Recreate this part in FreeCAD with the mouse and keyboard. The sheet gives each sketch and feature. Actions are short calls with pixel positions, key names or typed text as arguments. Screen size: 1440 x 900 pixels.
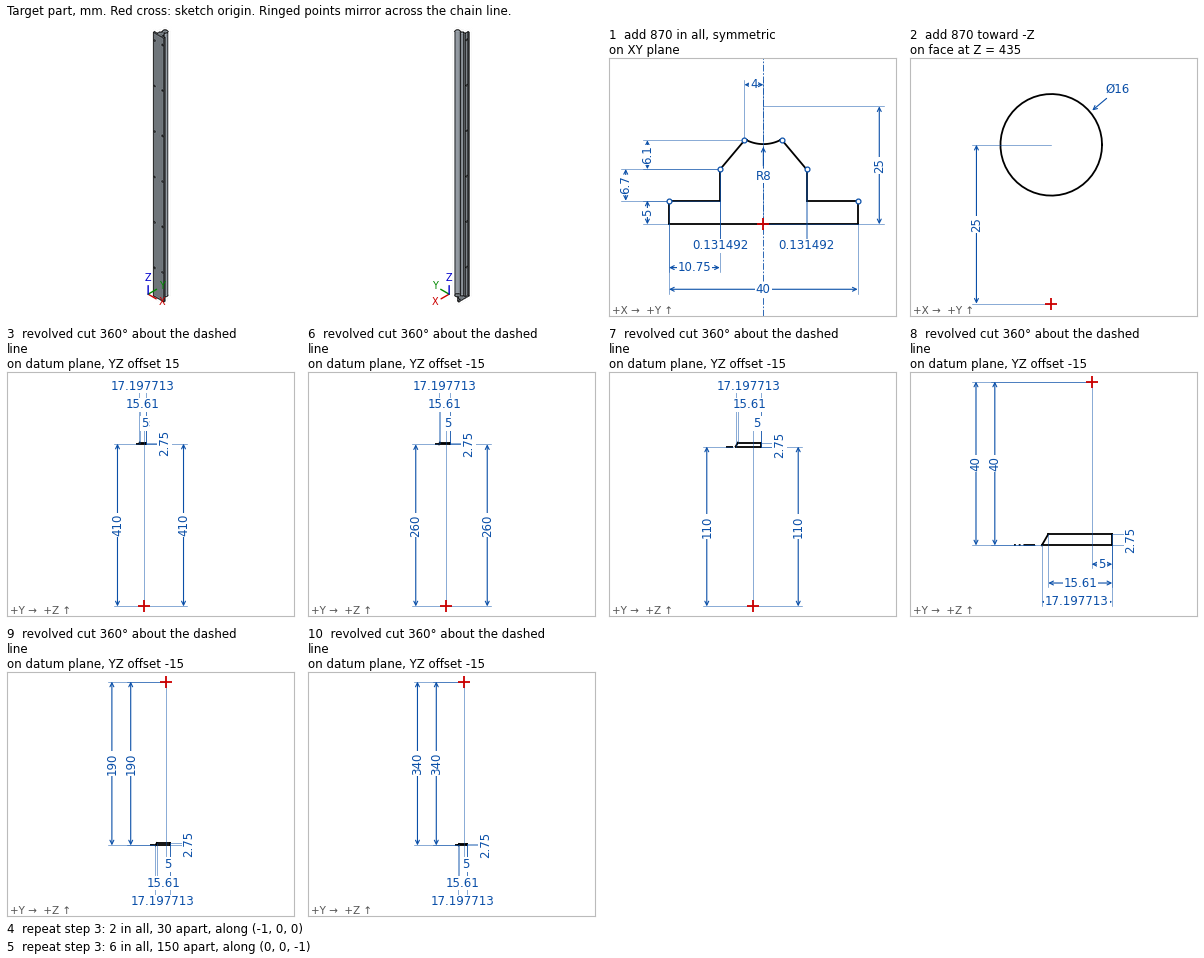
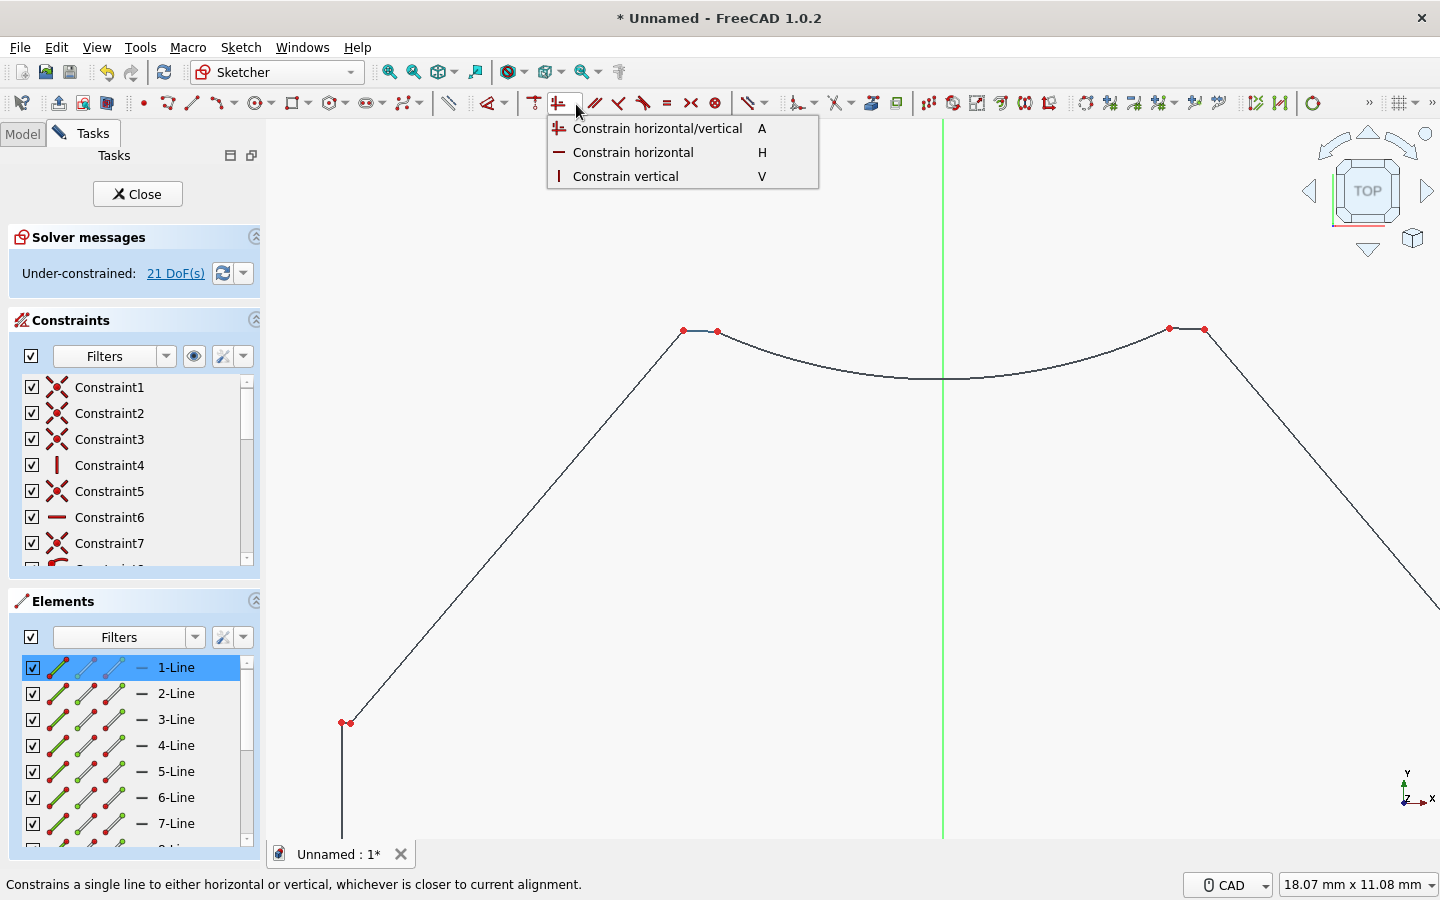
click(683, 152)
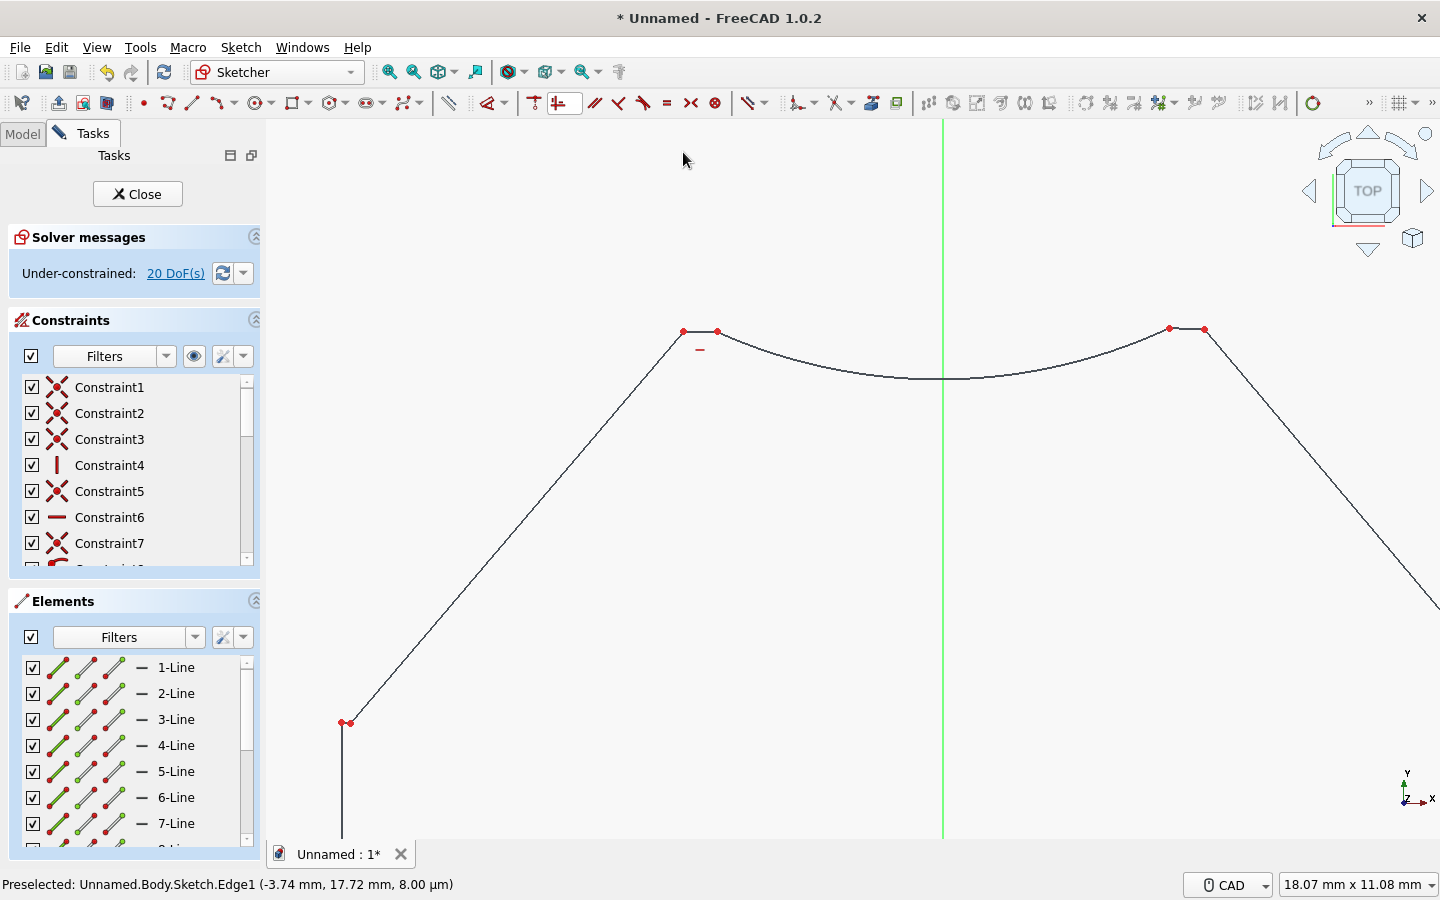
scroll(346, 723, up, 6)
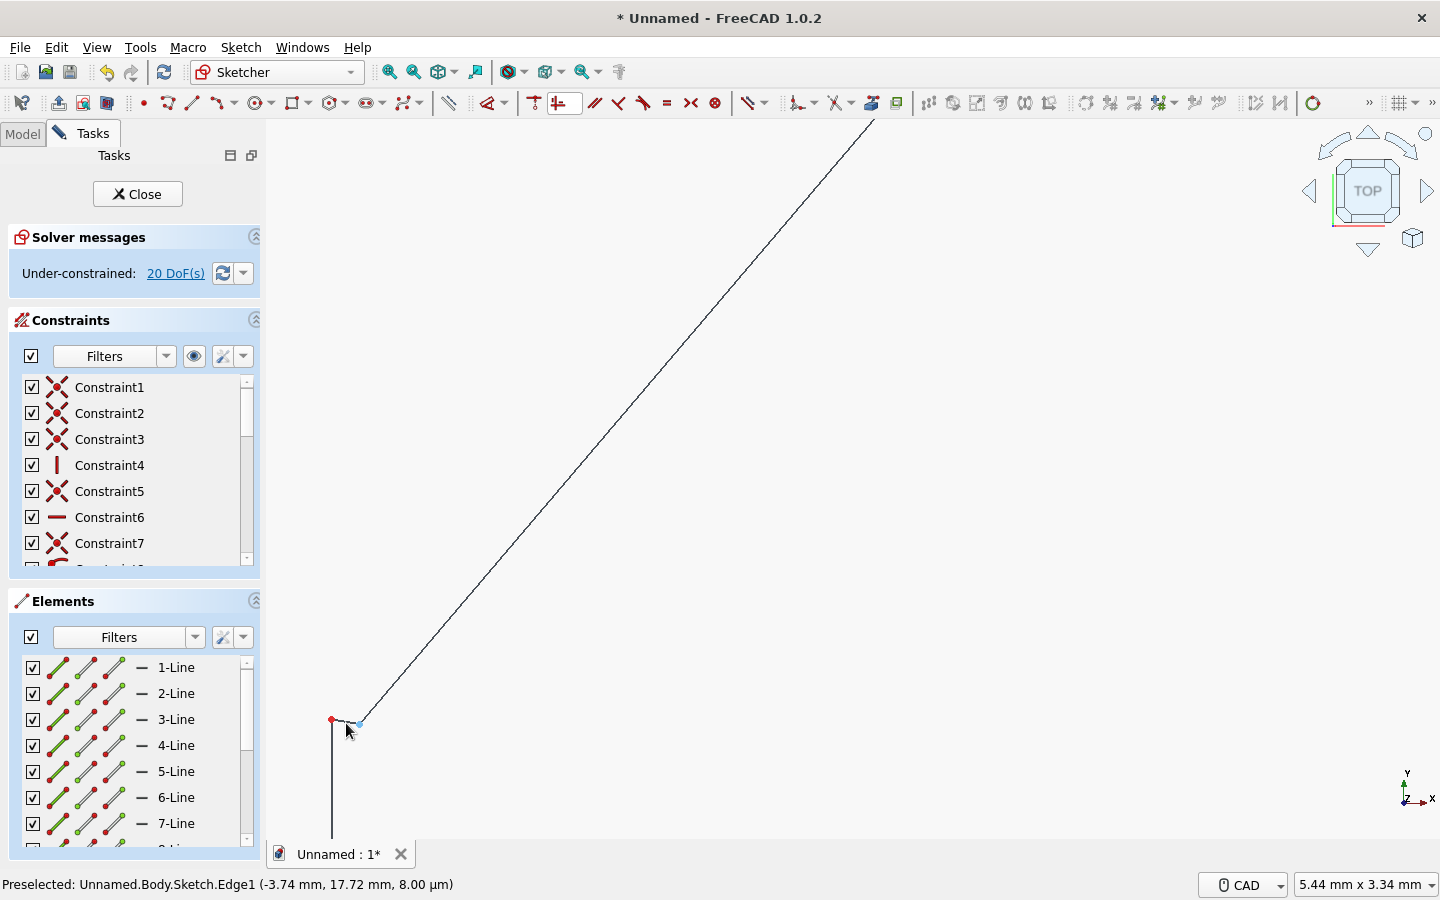
click(346, 722)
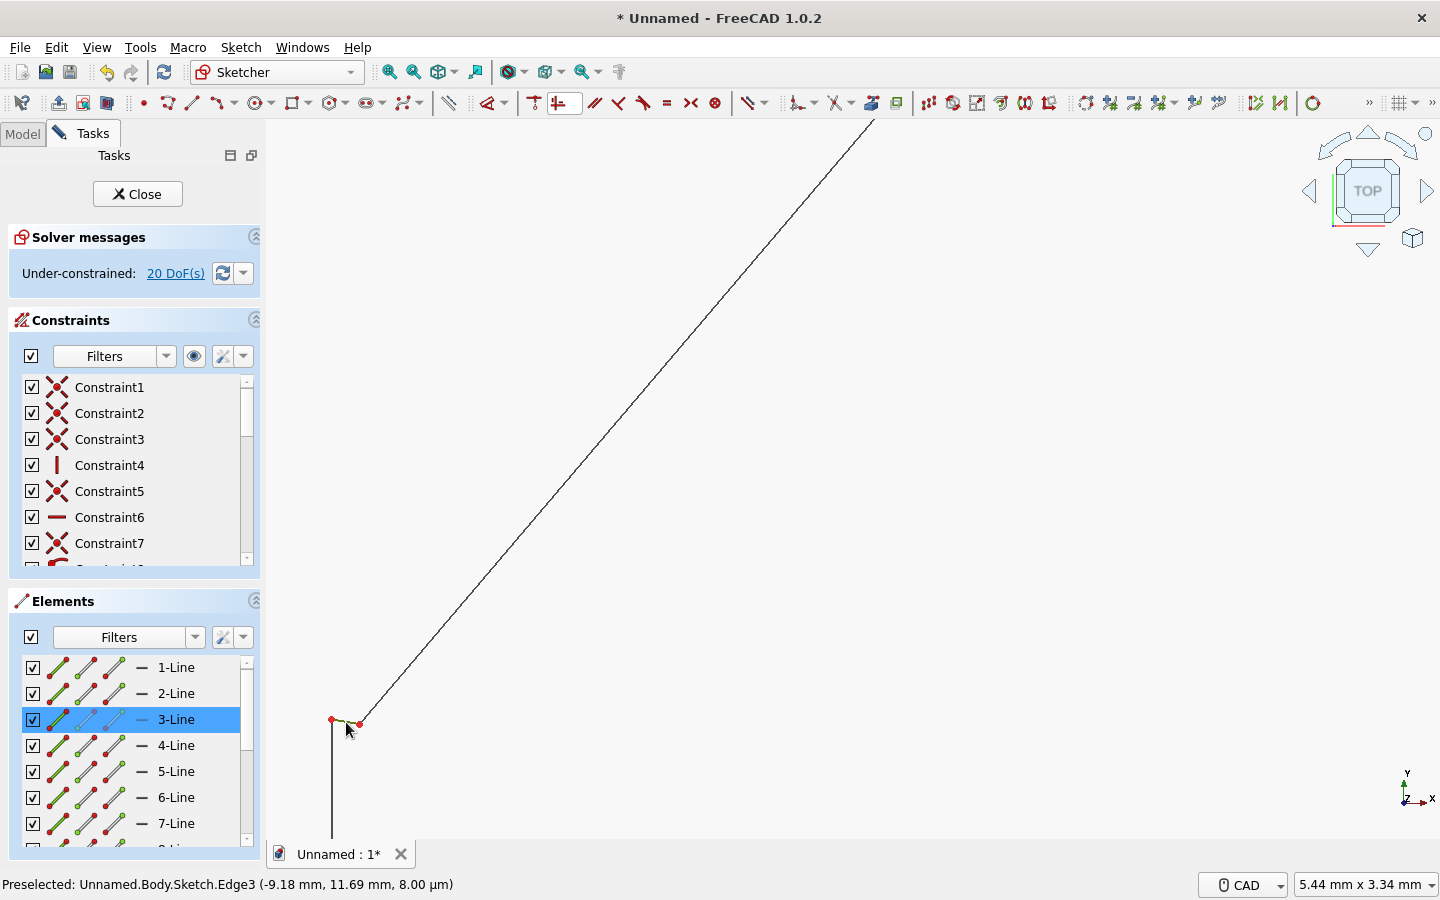
click(576, 104)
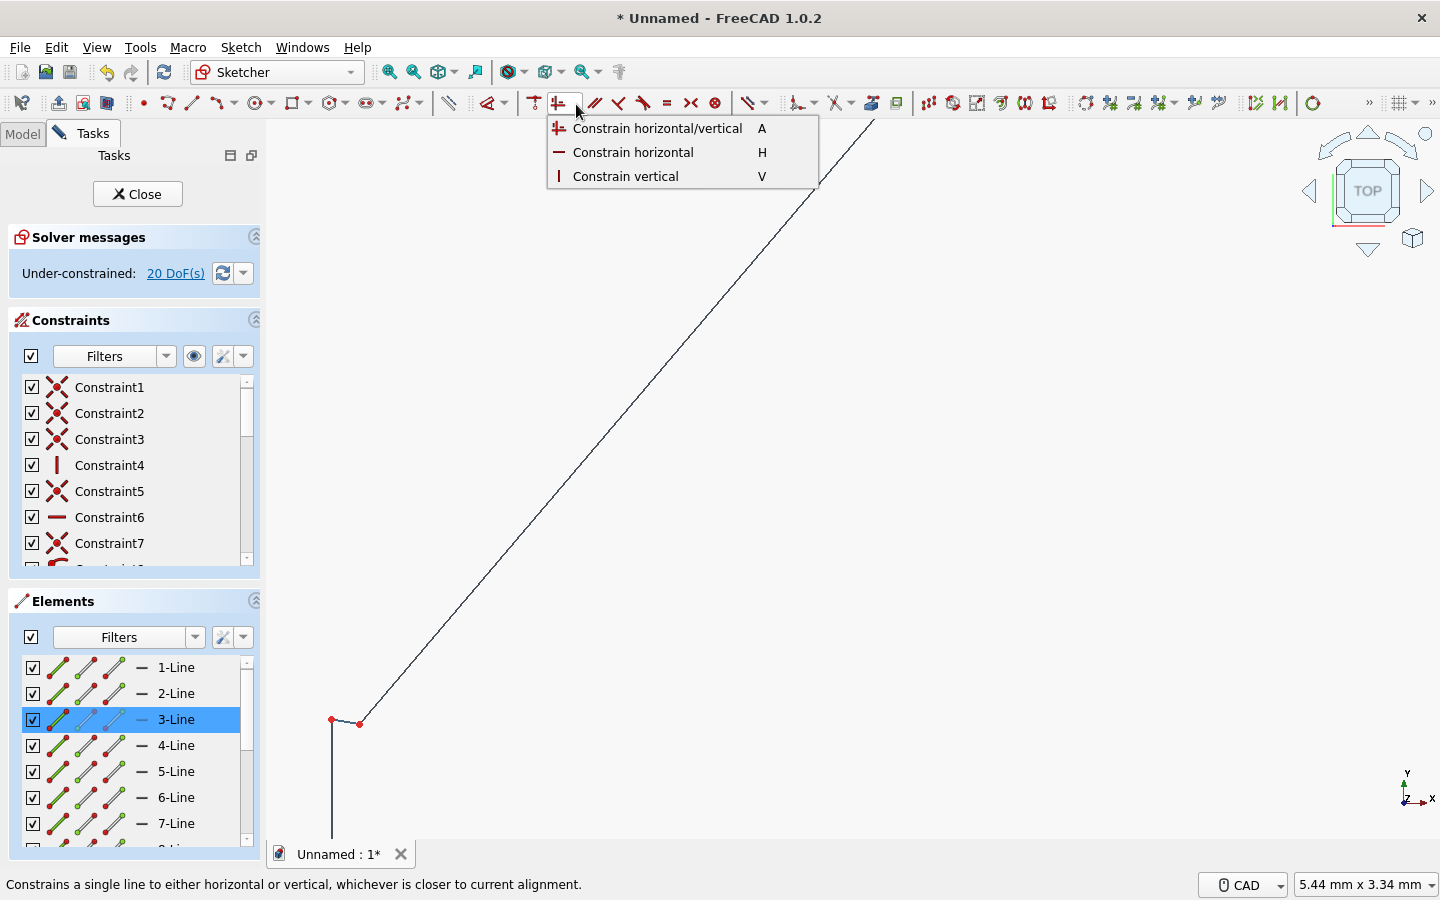
click(683, 152)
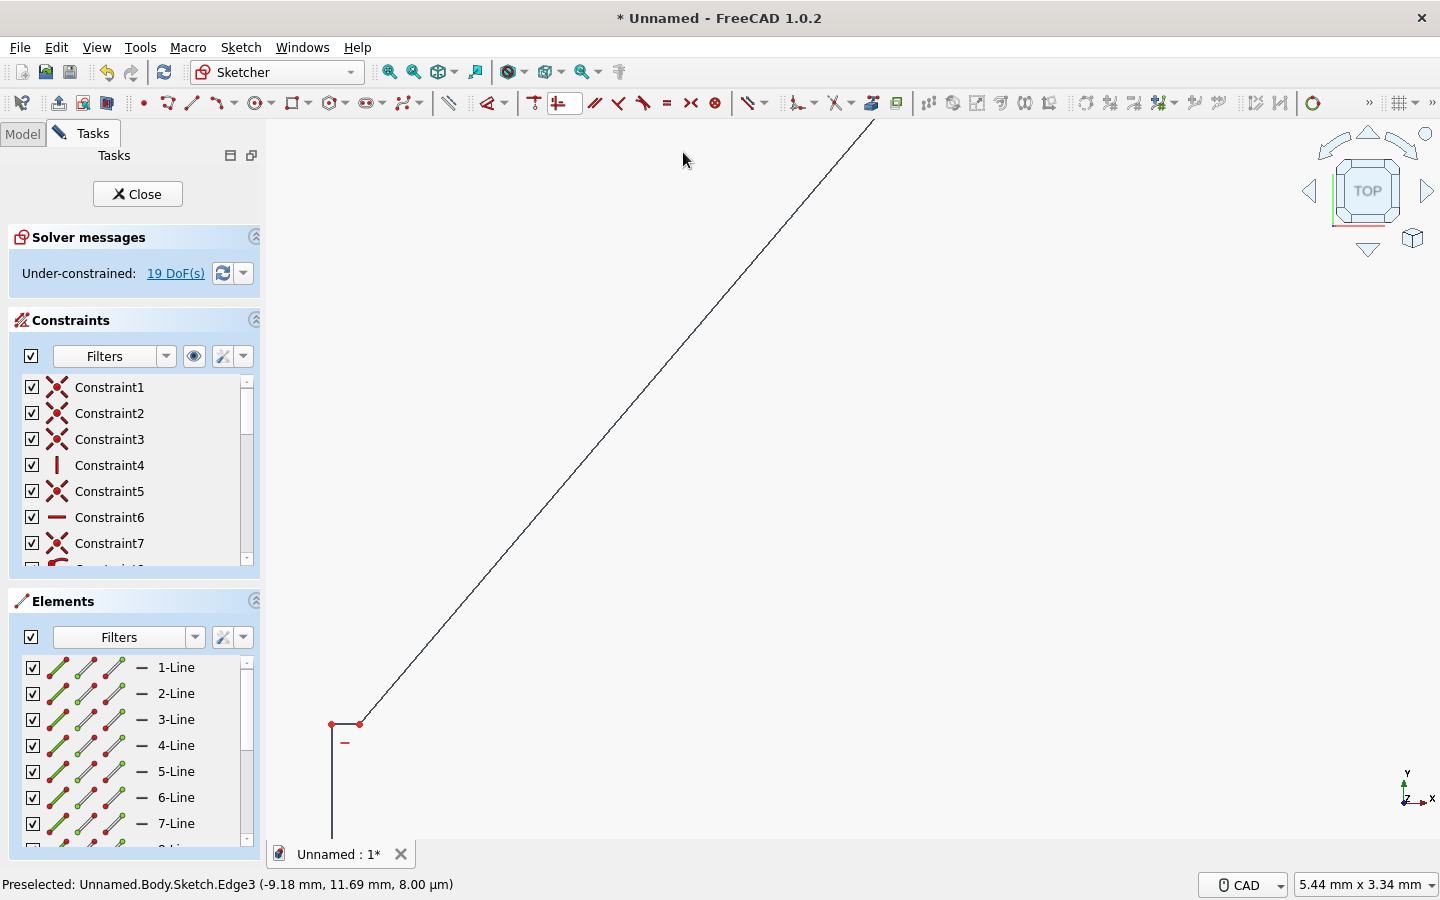
scroll(661, 411, down, 13)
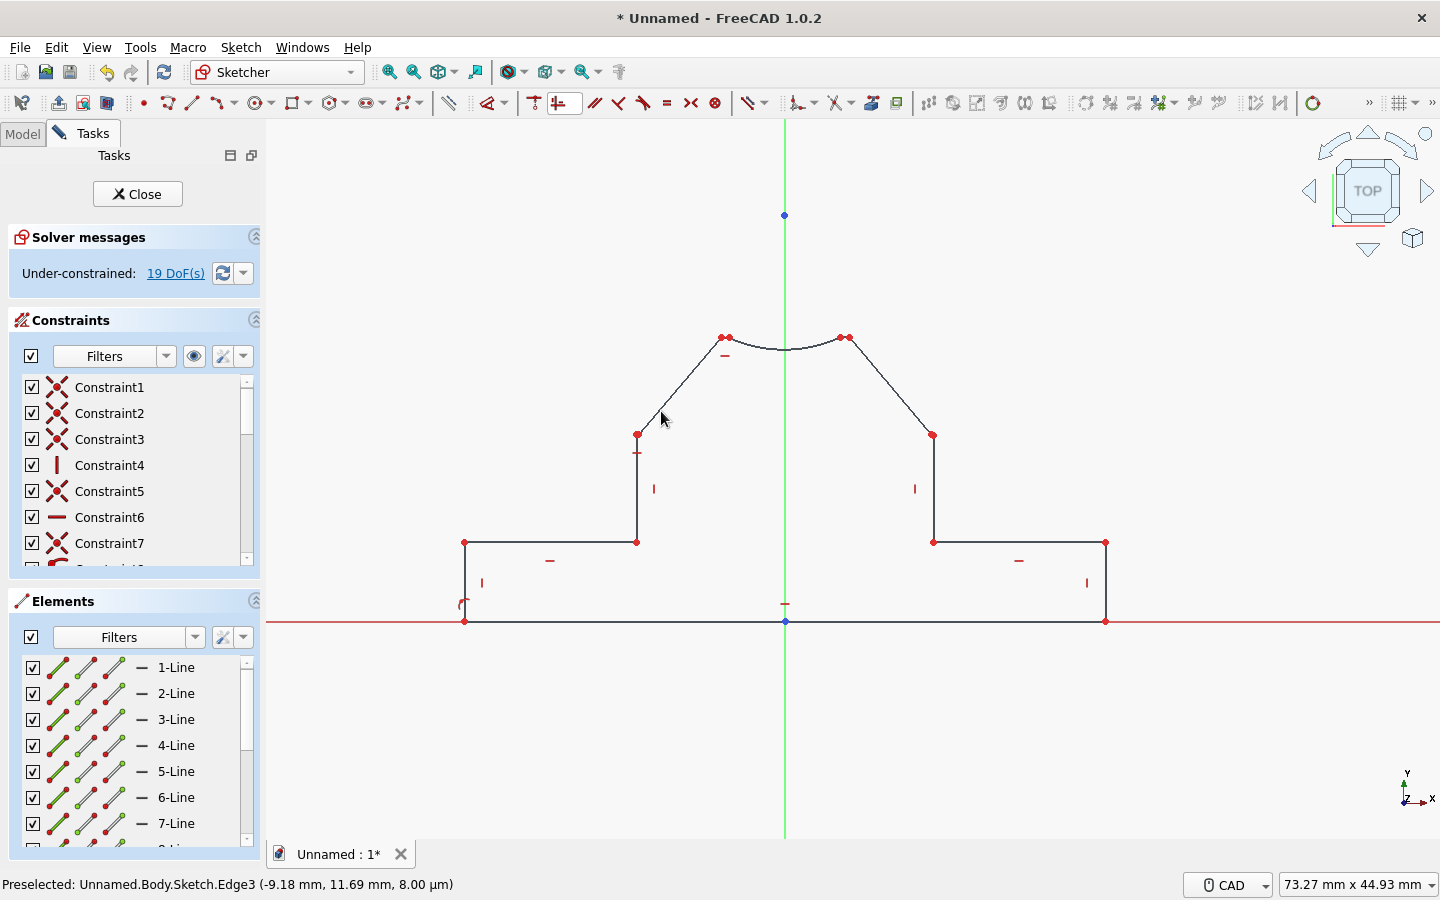
scroll(933, 435, up, 14)